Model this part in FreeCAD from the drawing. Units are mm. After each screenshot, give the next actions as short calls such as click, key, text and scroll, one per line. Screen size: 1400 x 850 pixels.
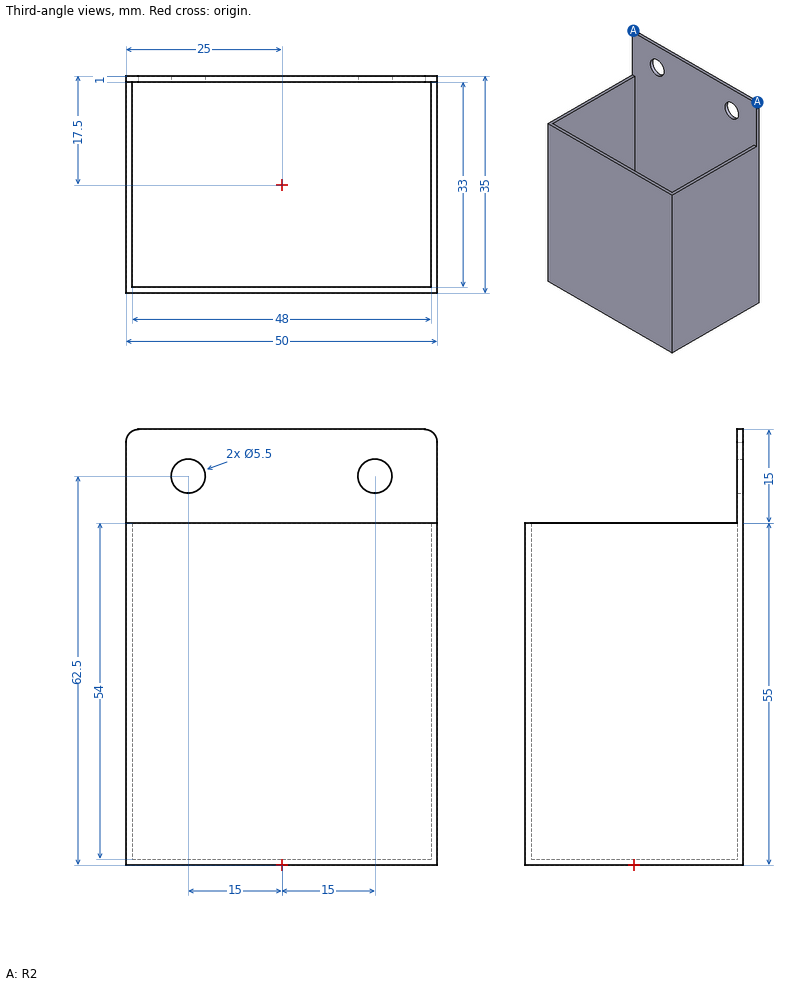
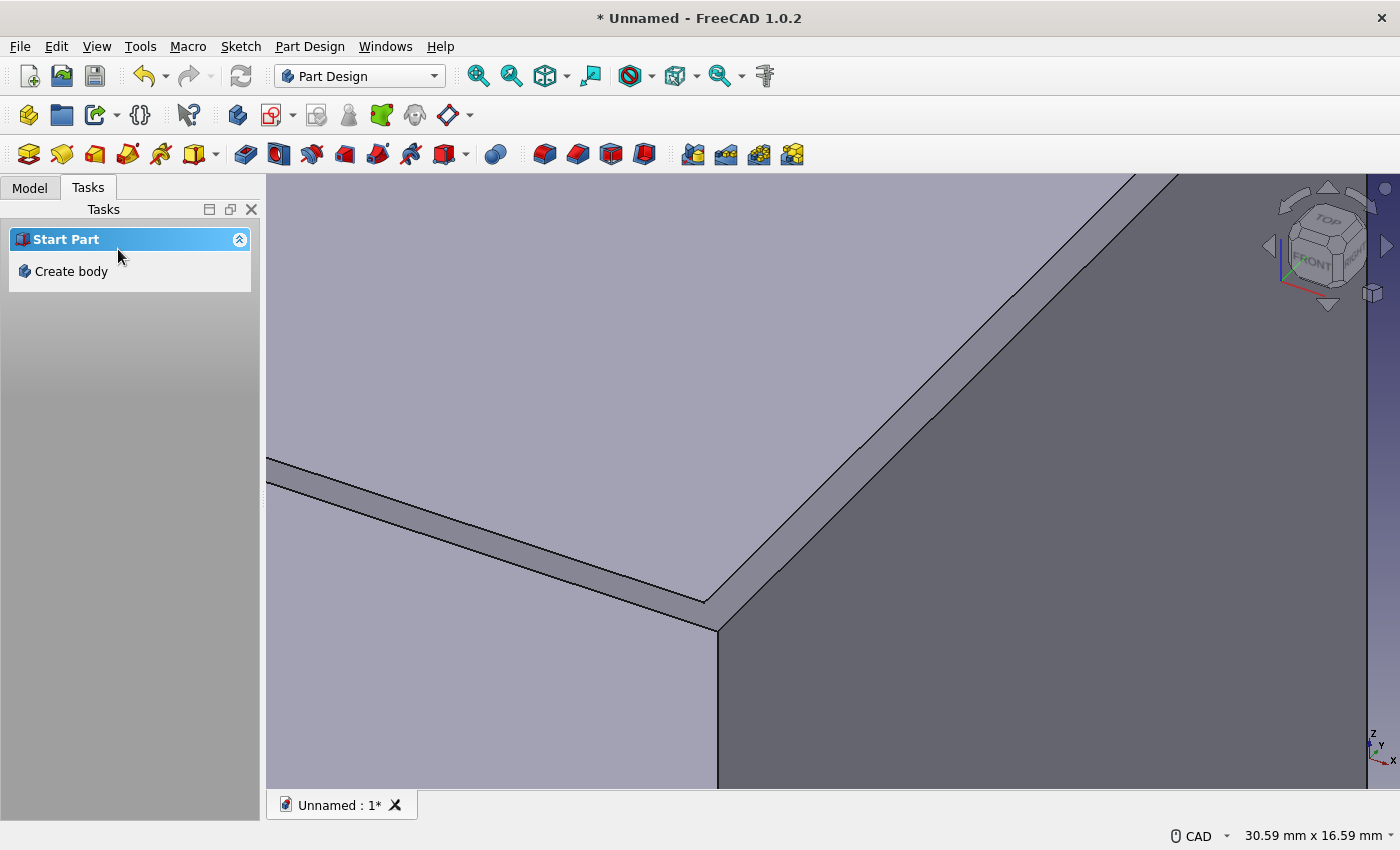
key(v)
key(f)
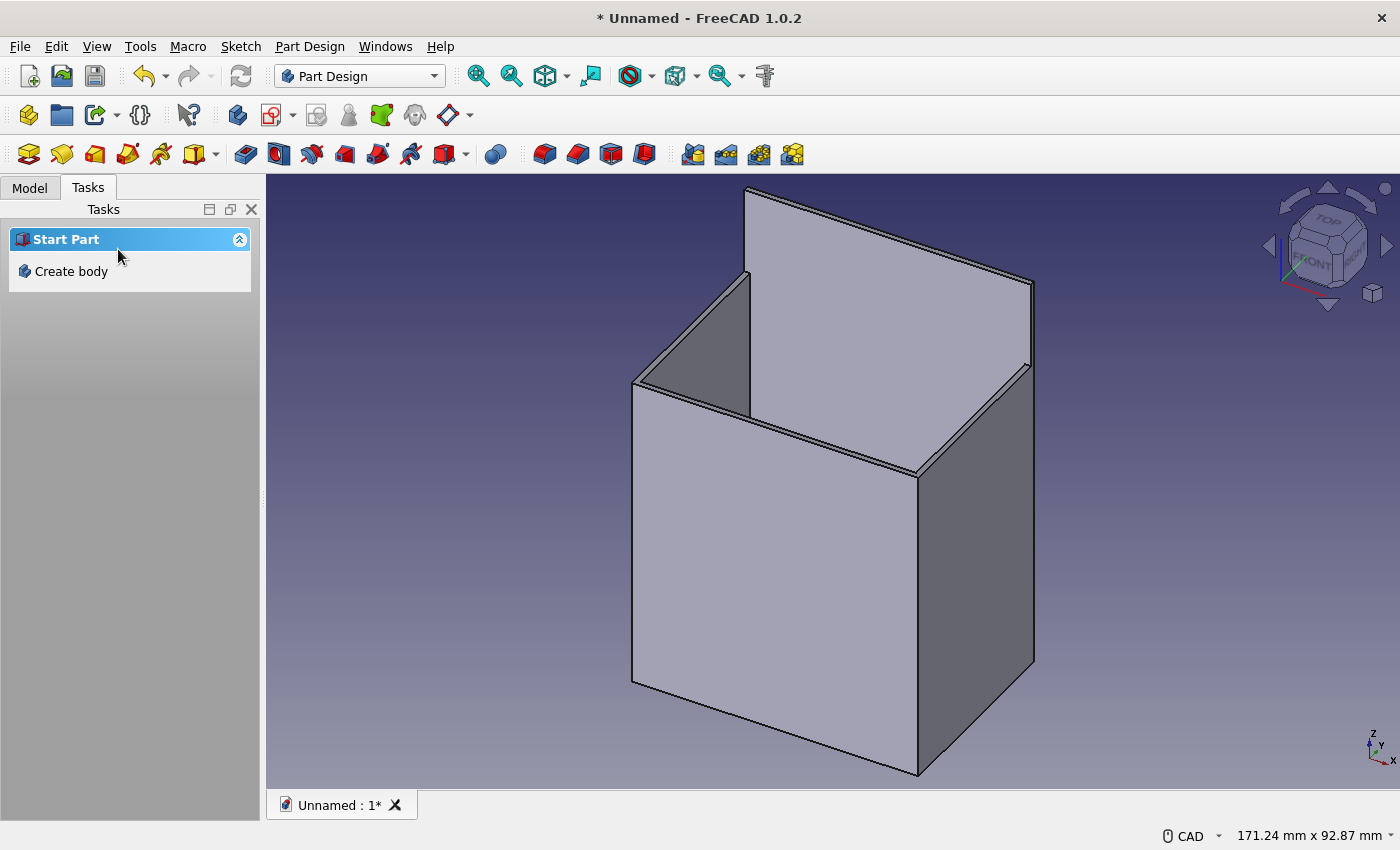
click(30, 188)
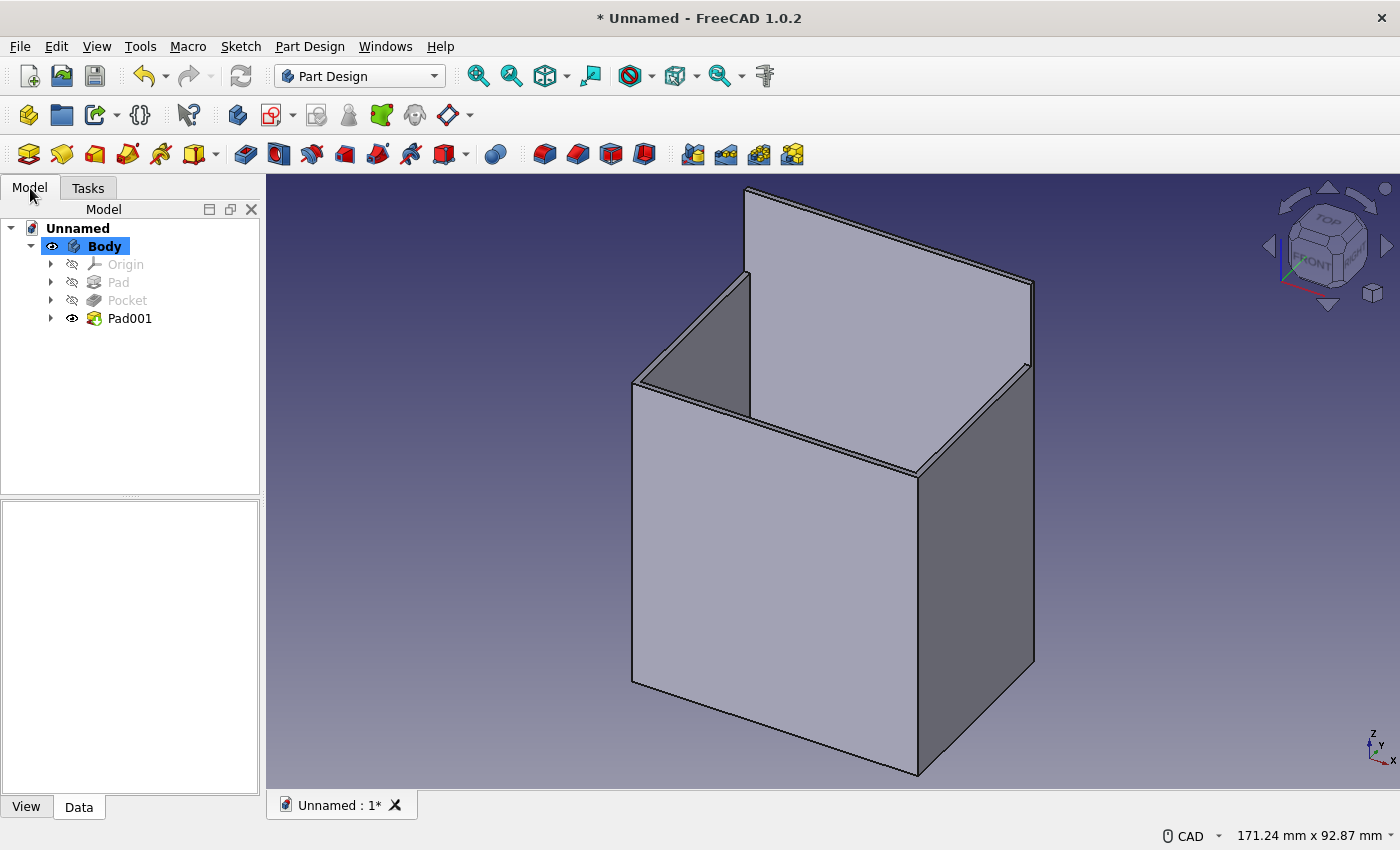
click(51, 264)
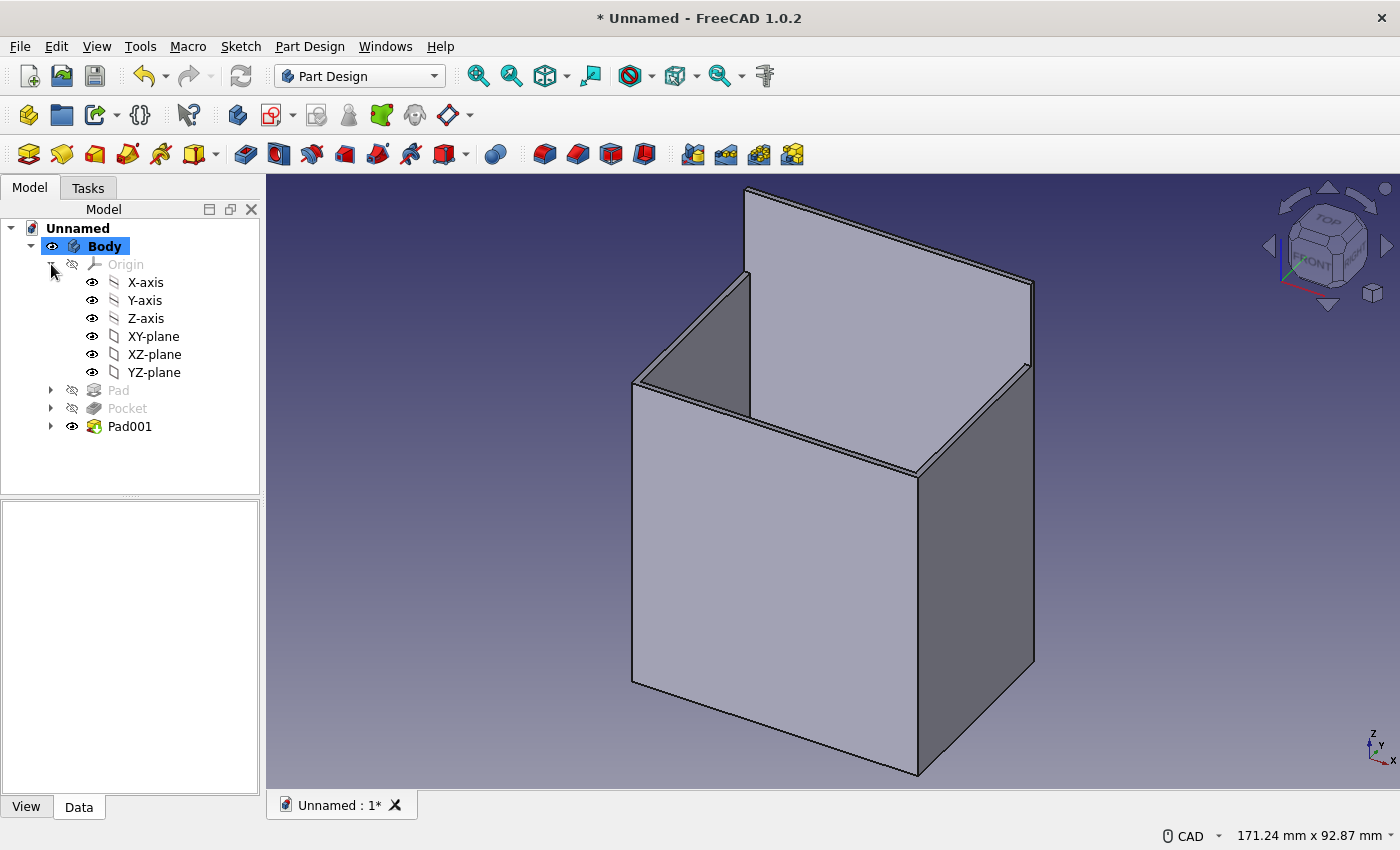
click(137, 354)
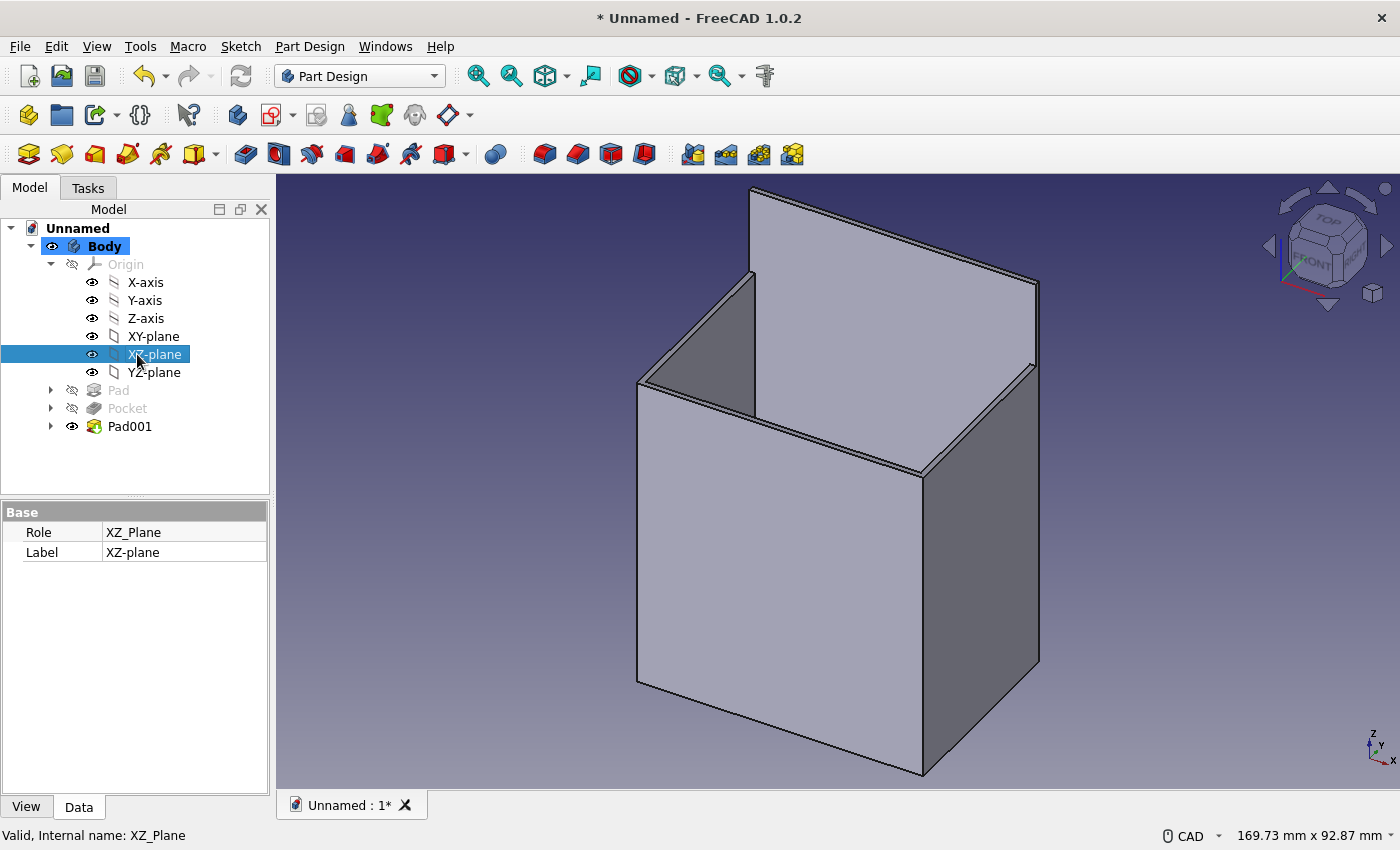
click(448, 116)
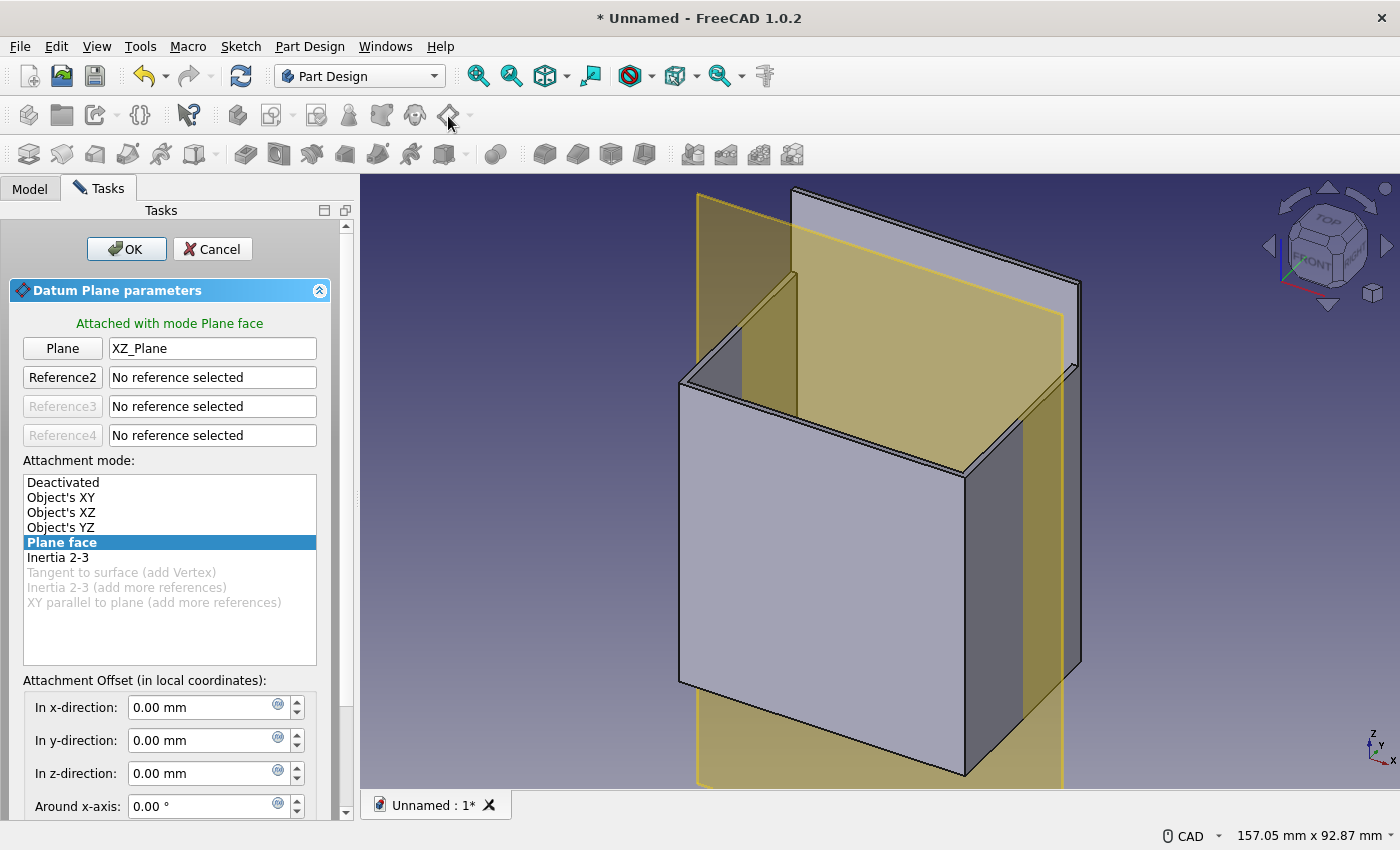
triple_click(210, 774)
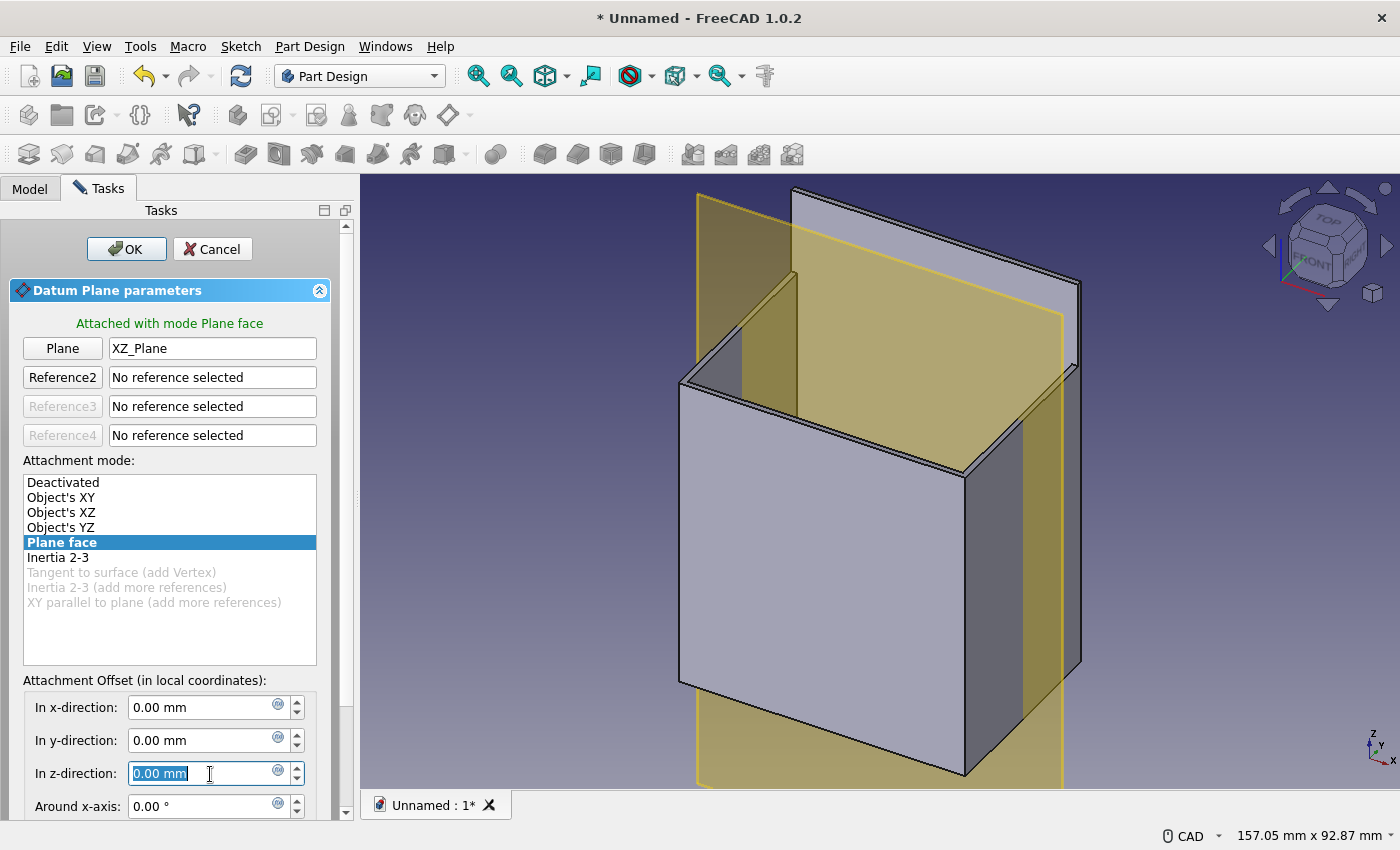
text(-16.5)
key(Tab)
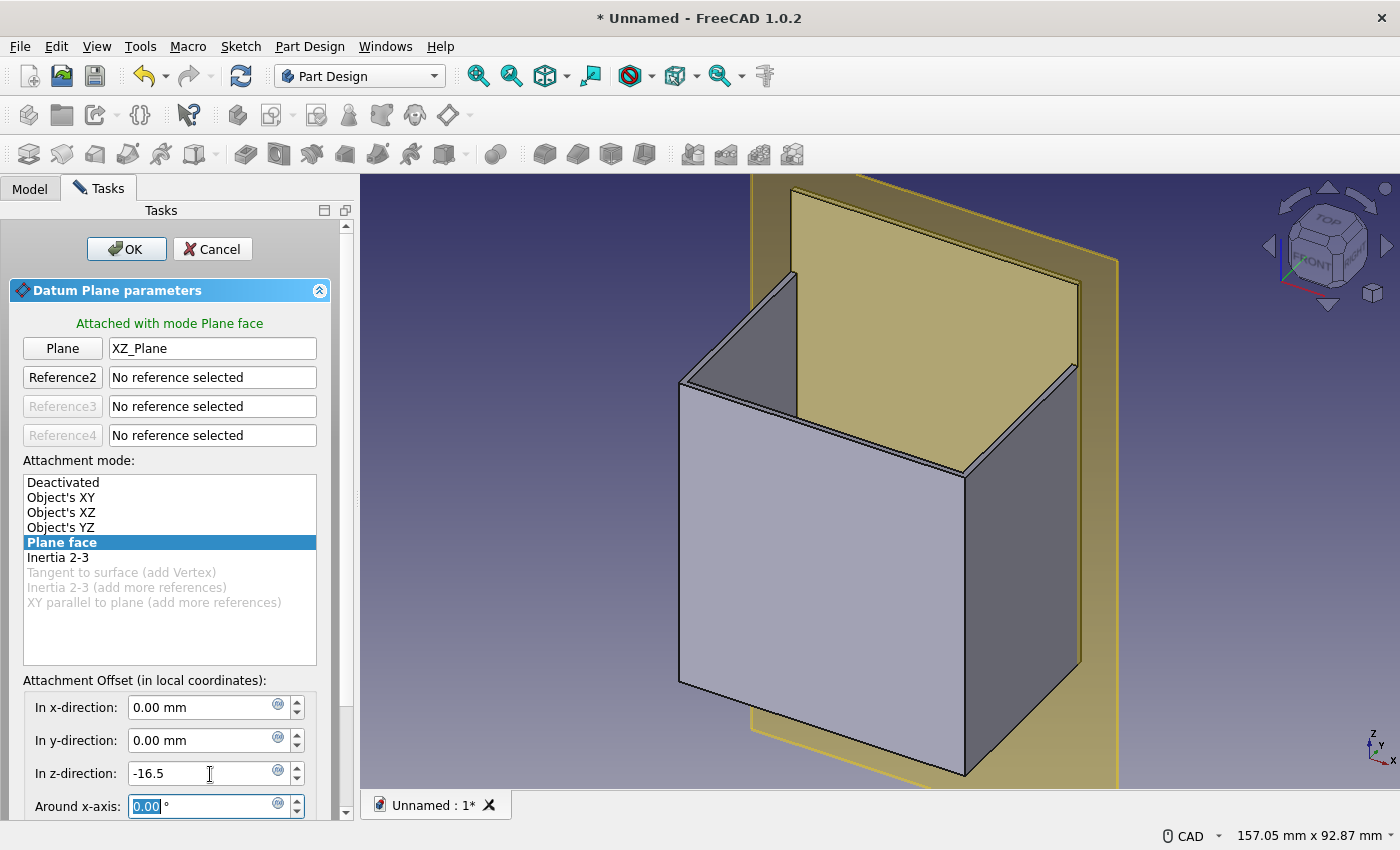
click(127, 249)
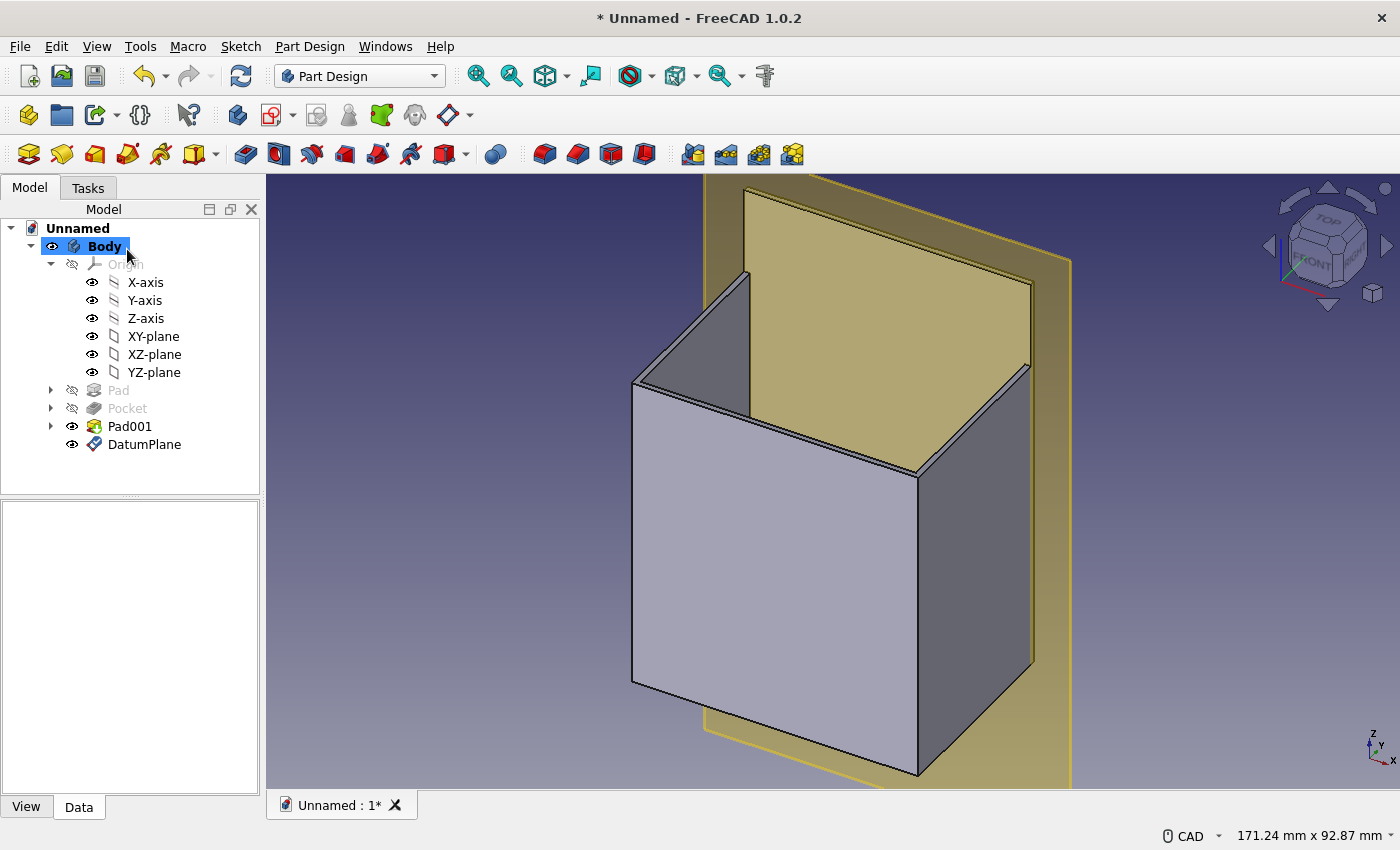
click(117, 444)